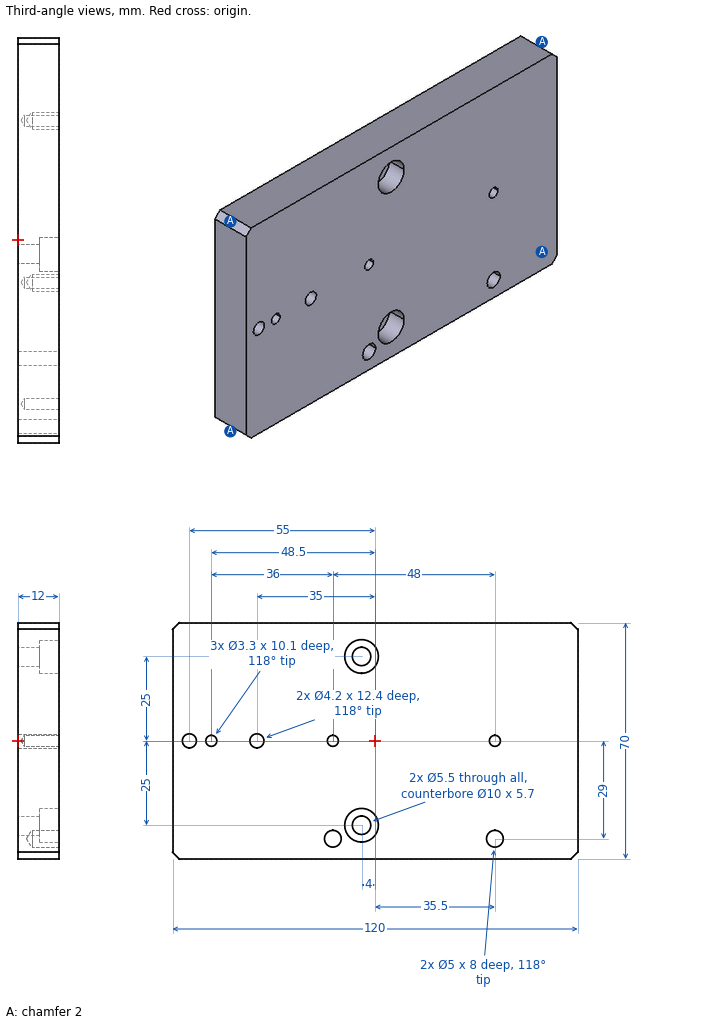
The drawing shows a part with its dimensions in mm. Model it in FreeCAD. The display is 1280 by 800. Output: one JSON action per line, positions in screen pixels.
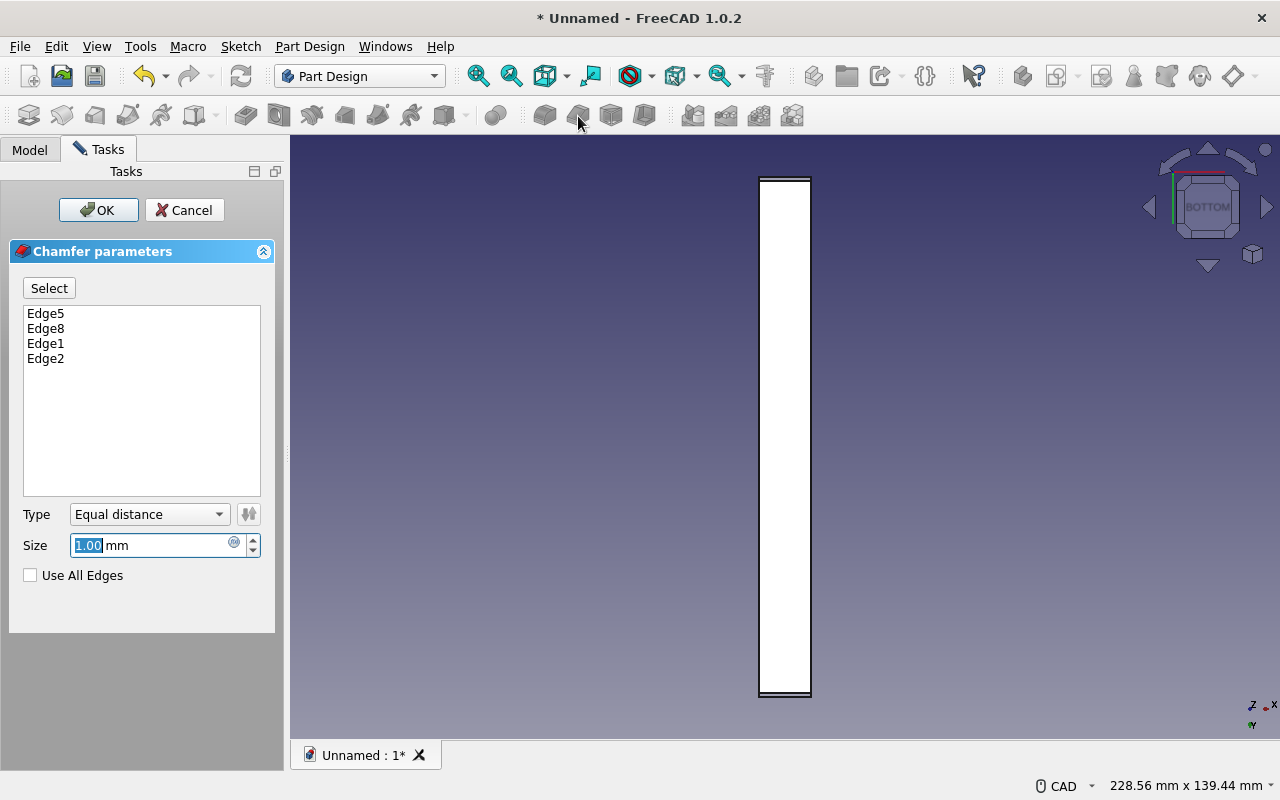
{"action": "type", "text": "2"}
{"action": "key", "text": "Tab"}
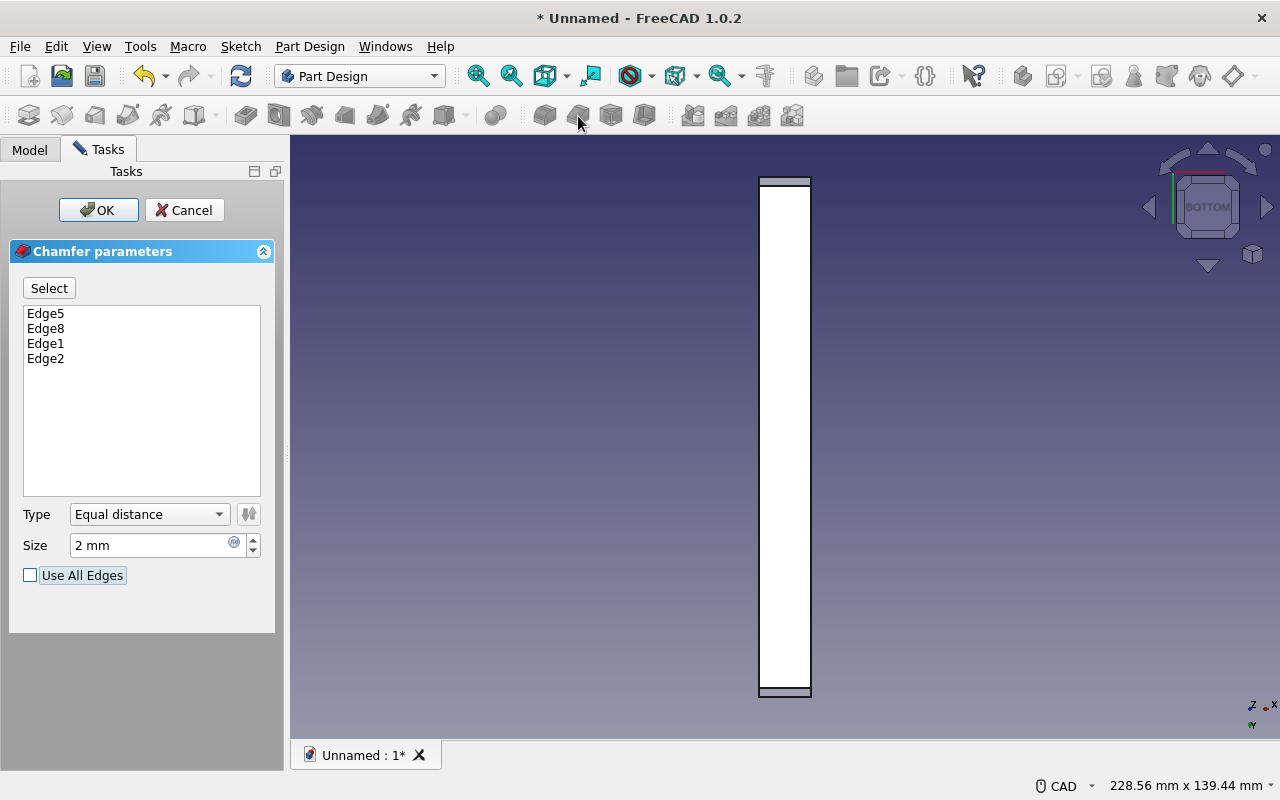
{"action": "left_click", "coordinate": [99, 210]}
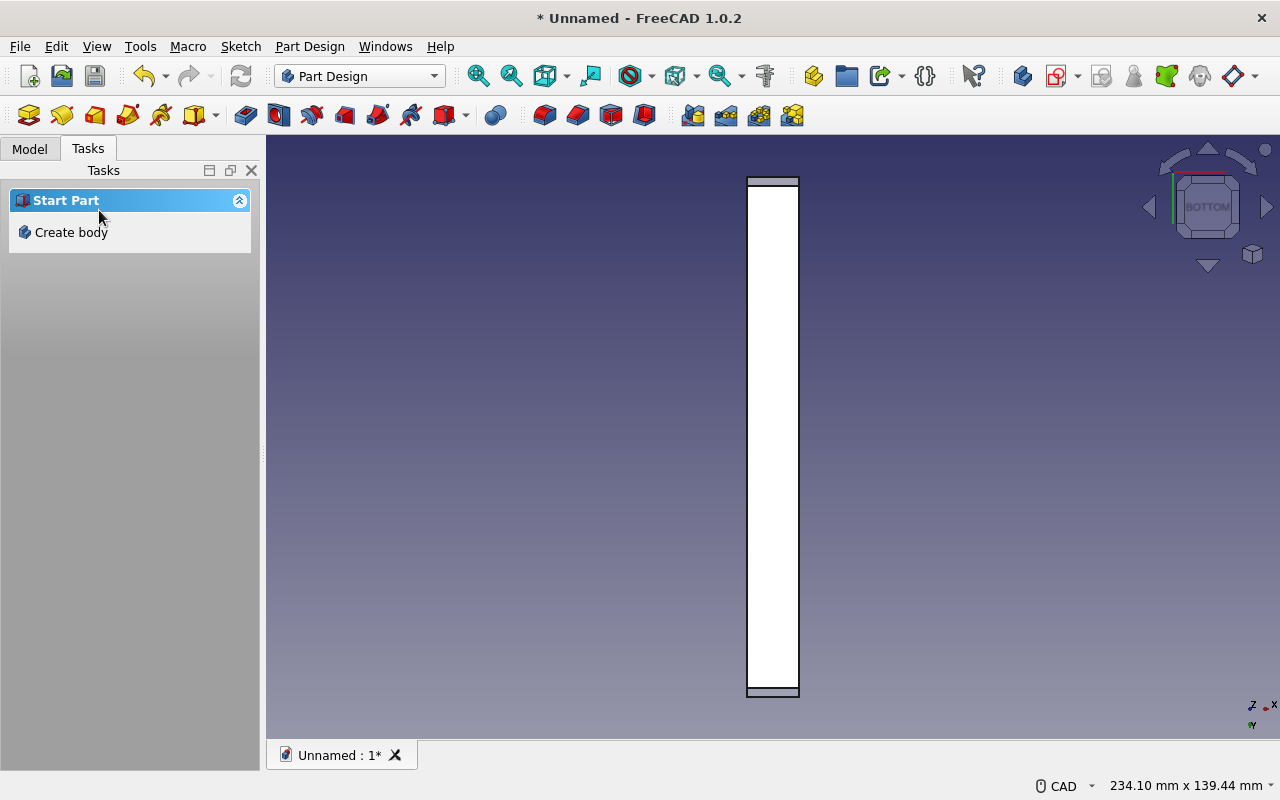
{"action": "key", "text": "0"}